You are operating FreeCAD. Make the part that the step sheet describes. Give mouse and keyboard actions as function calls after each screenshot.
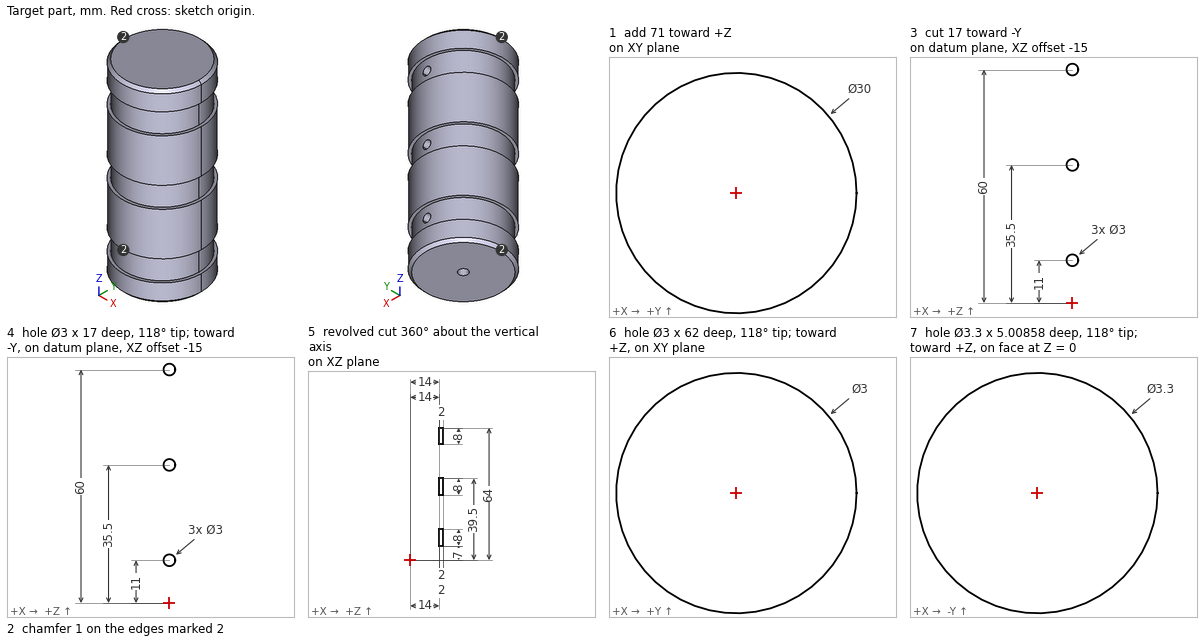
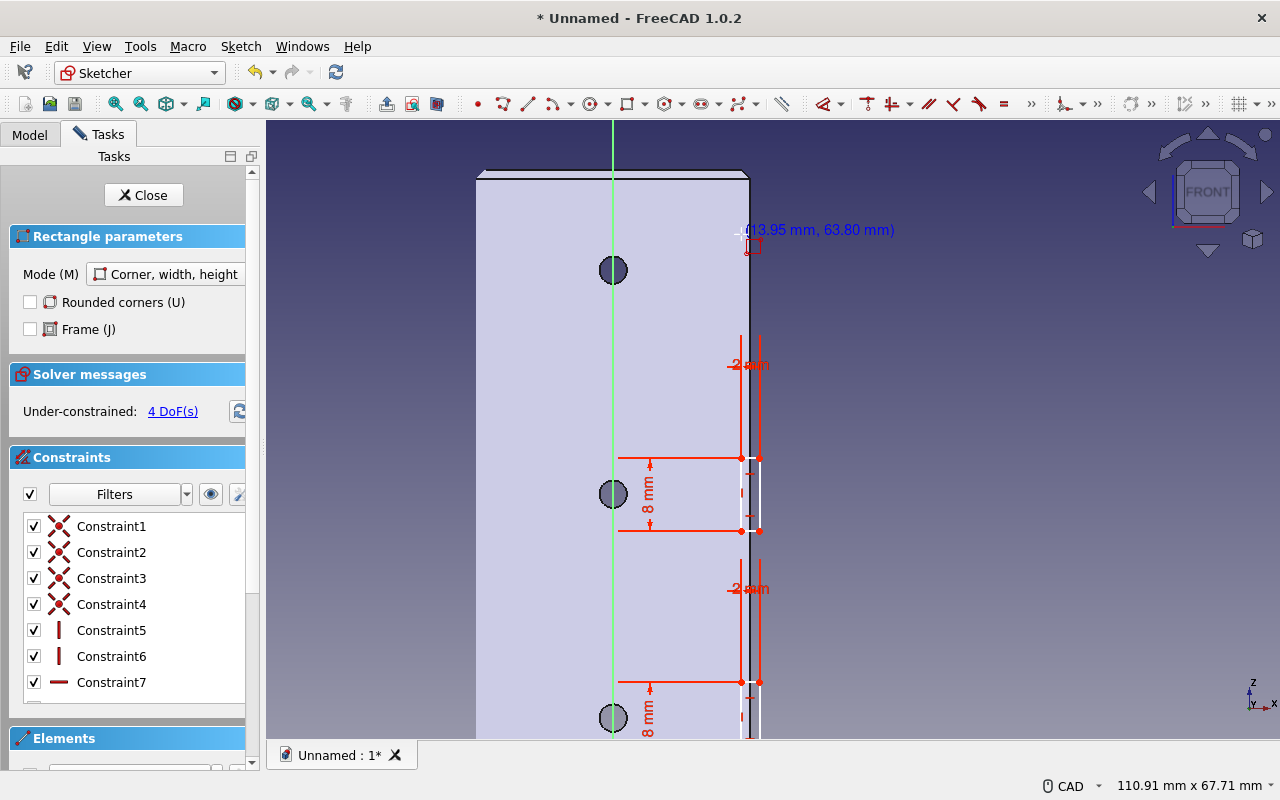
click(741, 234)
move(759, 307)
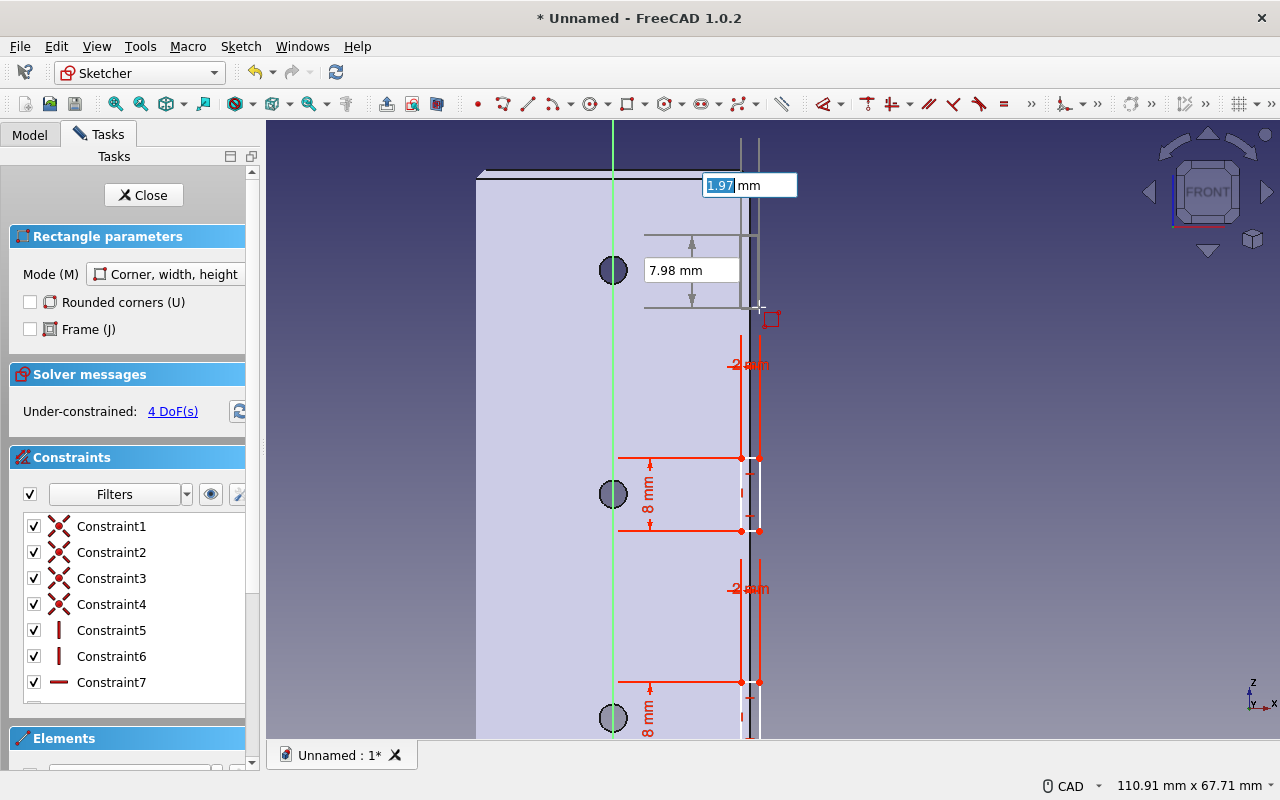
text(2)
key(Tab)
text(8)
key(Return)
key(Escape)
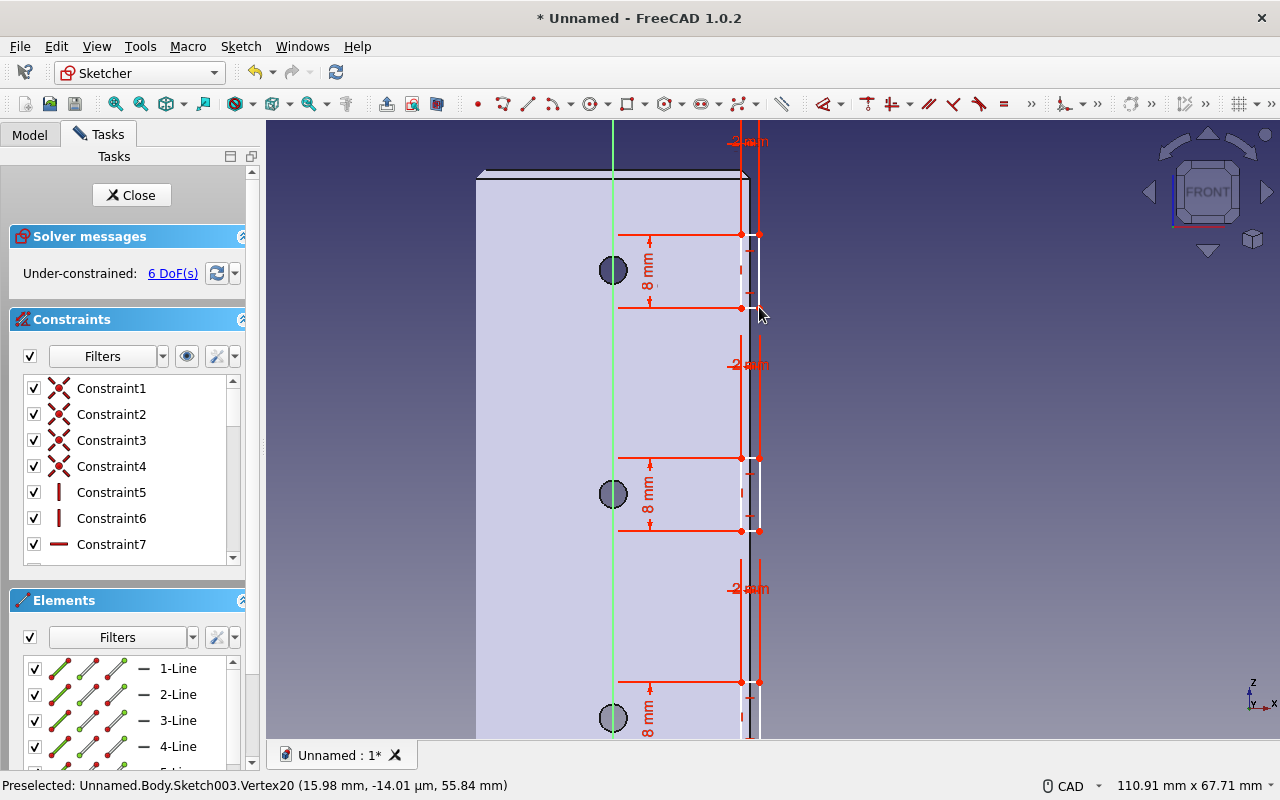
click(822, 104)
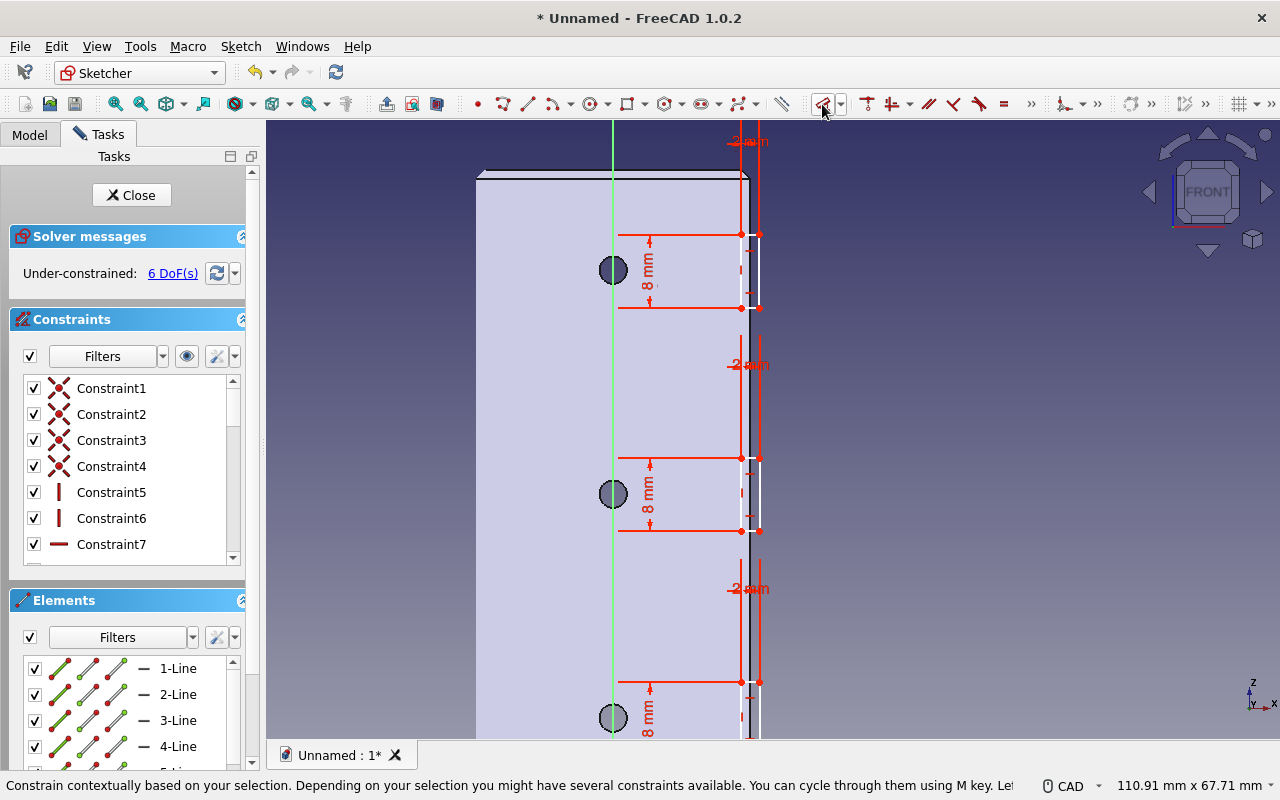
scroll(741, 233, down, 2)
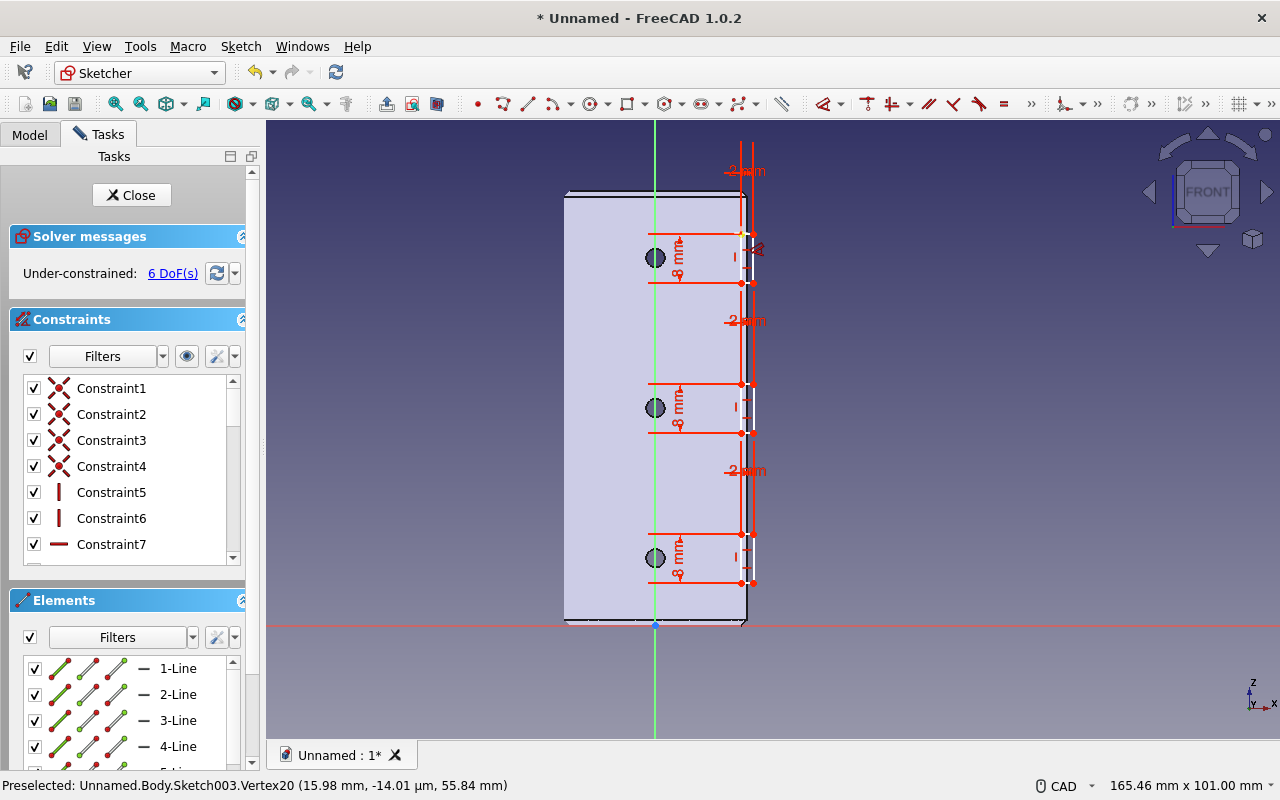
click(741, 583)
click(621, 604)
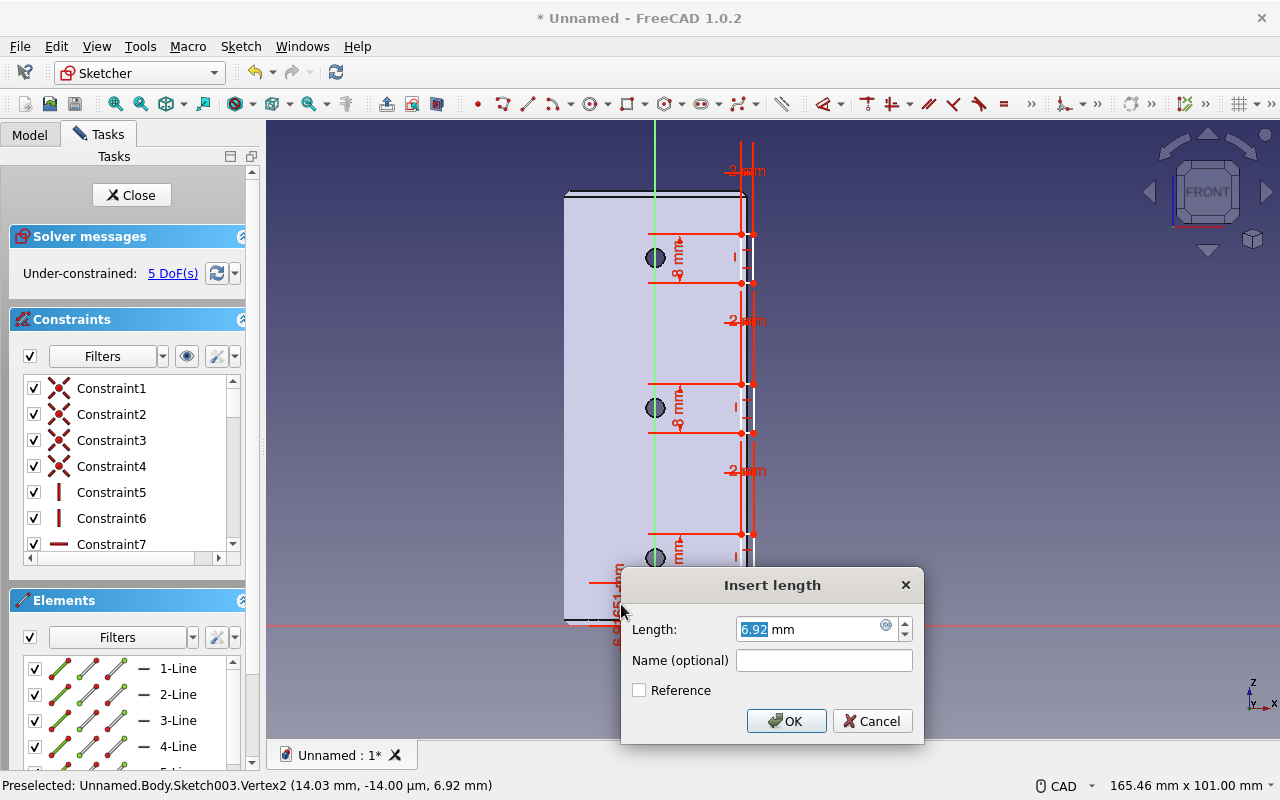
text(7)
key(Return)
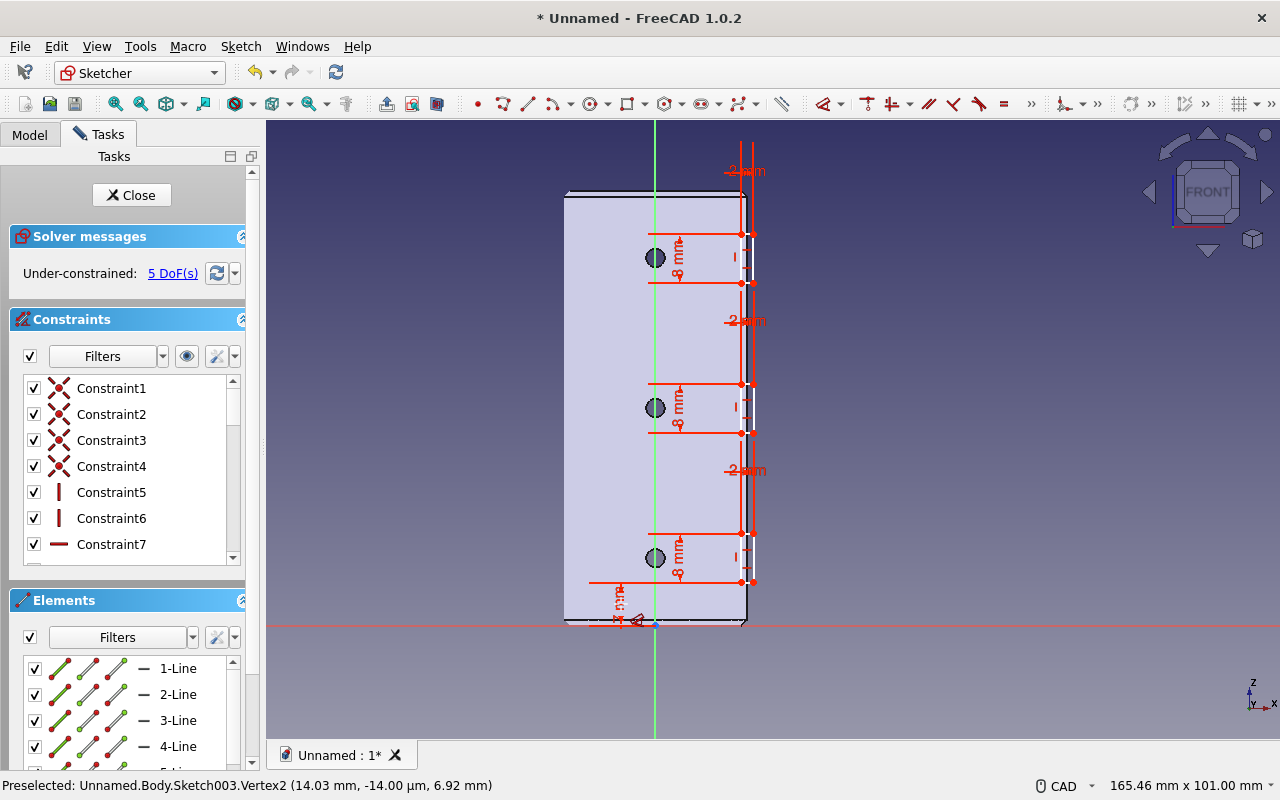
click(741, 534)
click(698, 660)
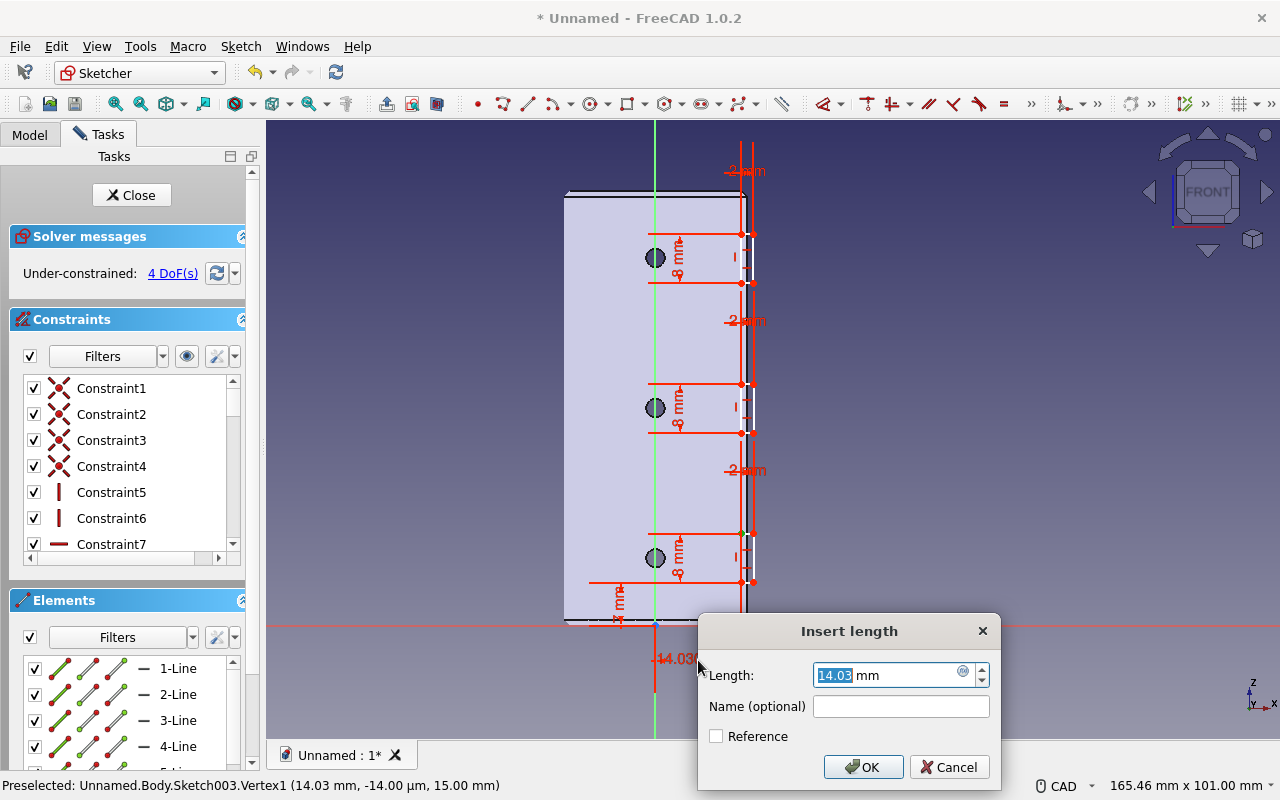
text(14)
key(Return)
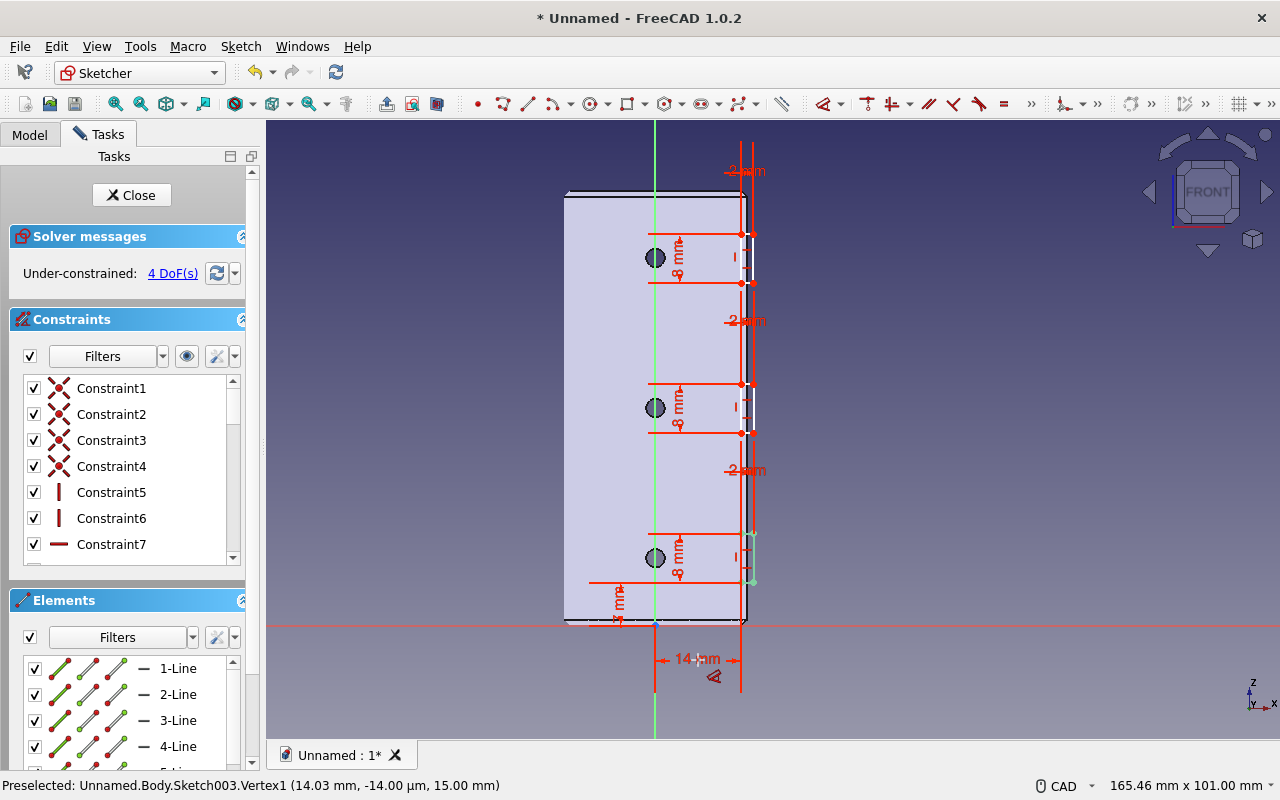
click(741, 384)
click(698, 350)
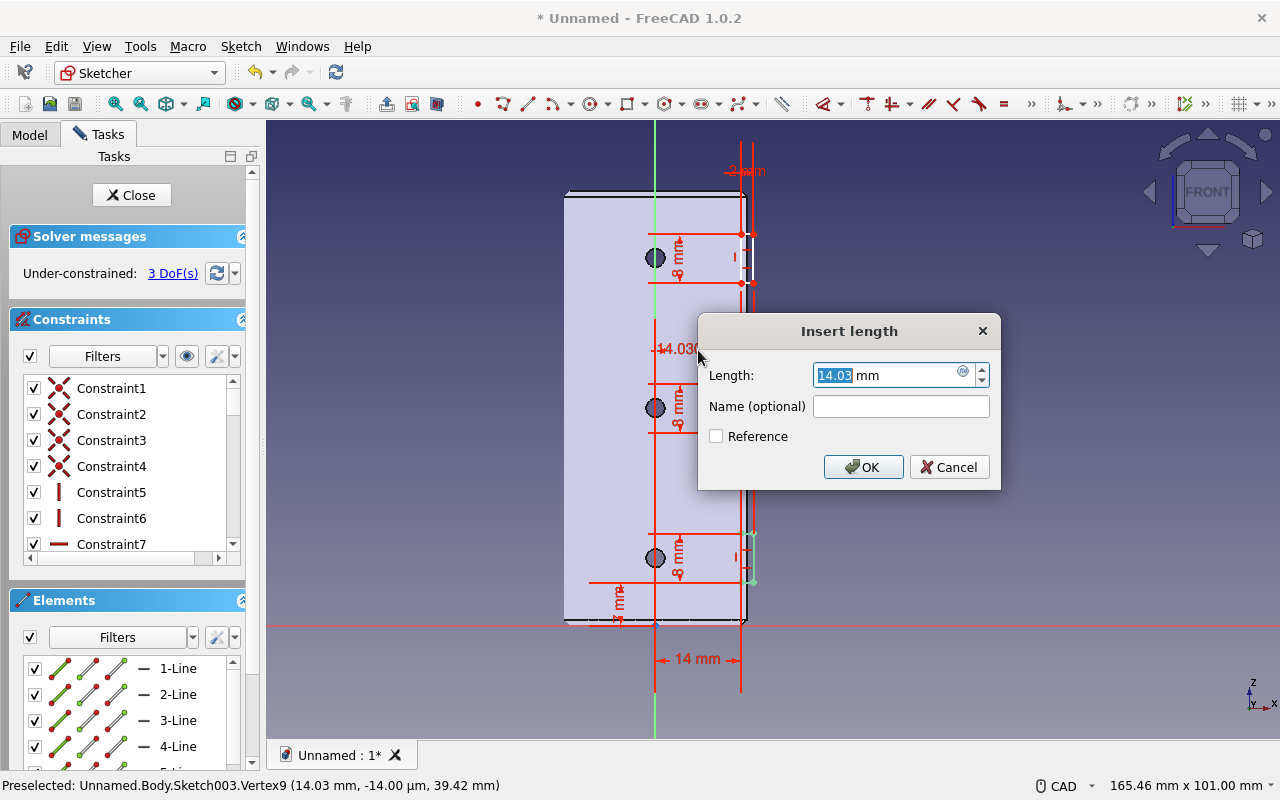
text(14)
key(Return)